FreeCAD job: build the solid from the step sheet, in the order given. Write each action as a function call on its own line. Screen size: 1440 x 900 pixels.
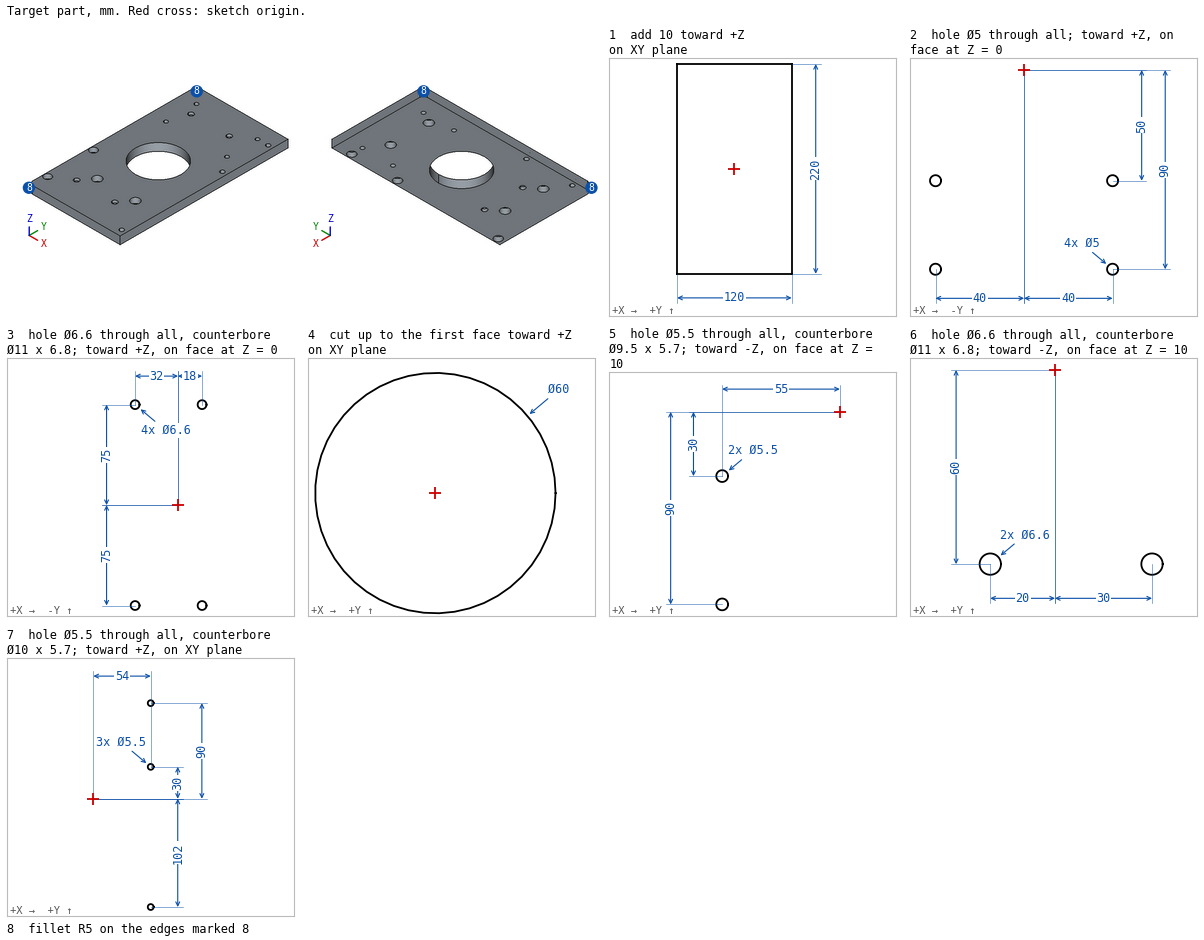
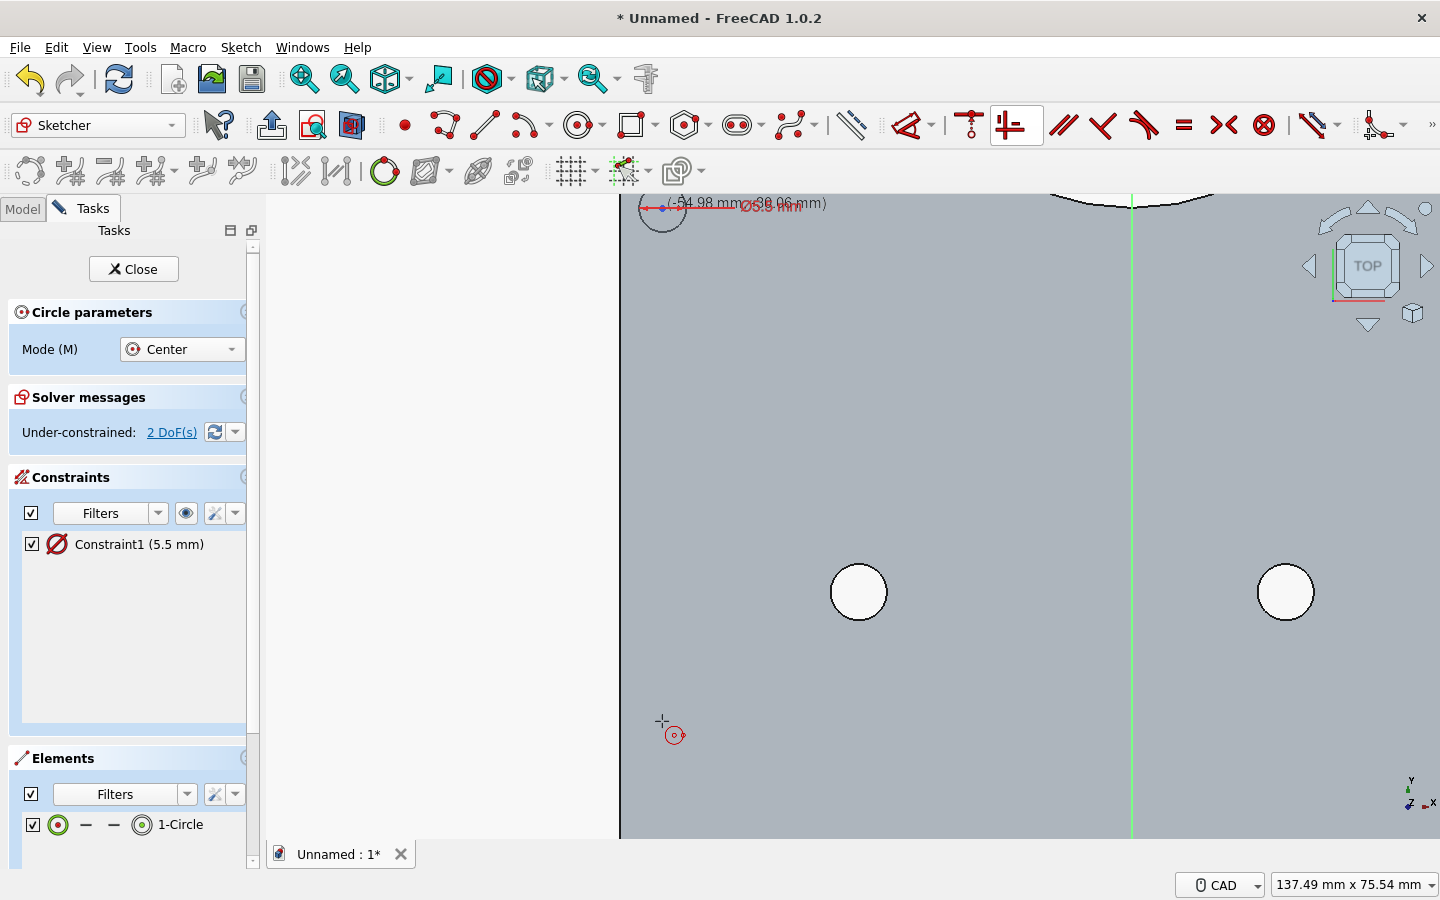
click(662, 720)
move(679, 704)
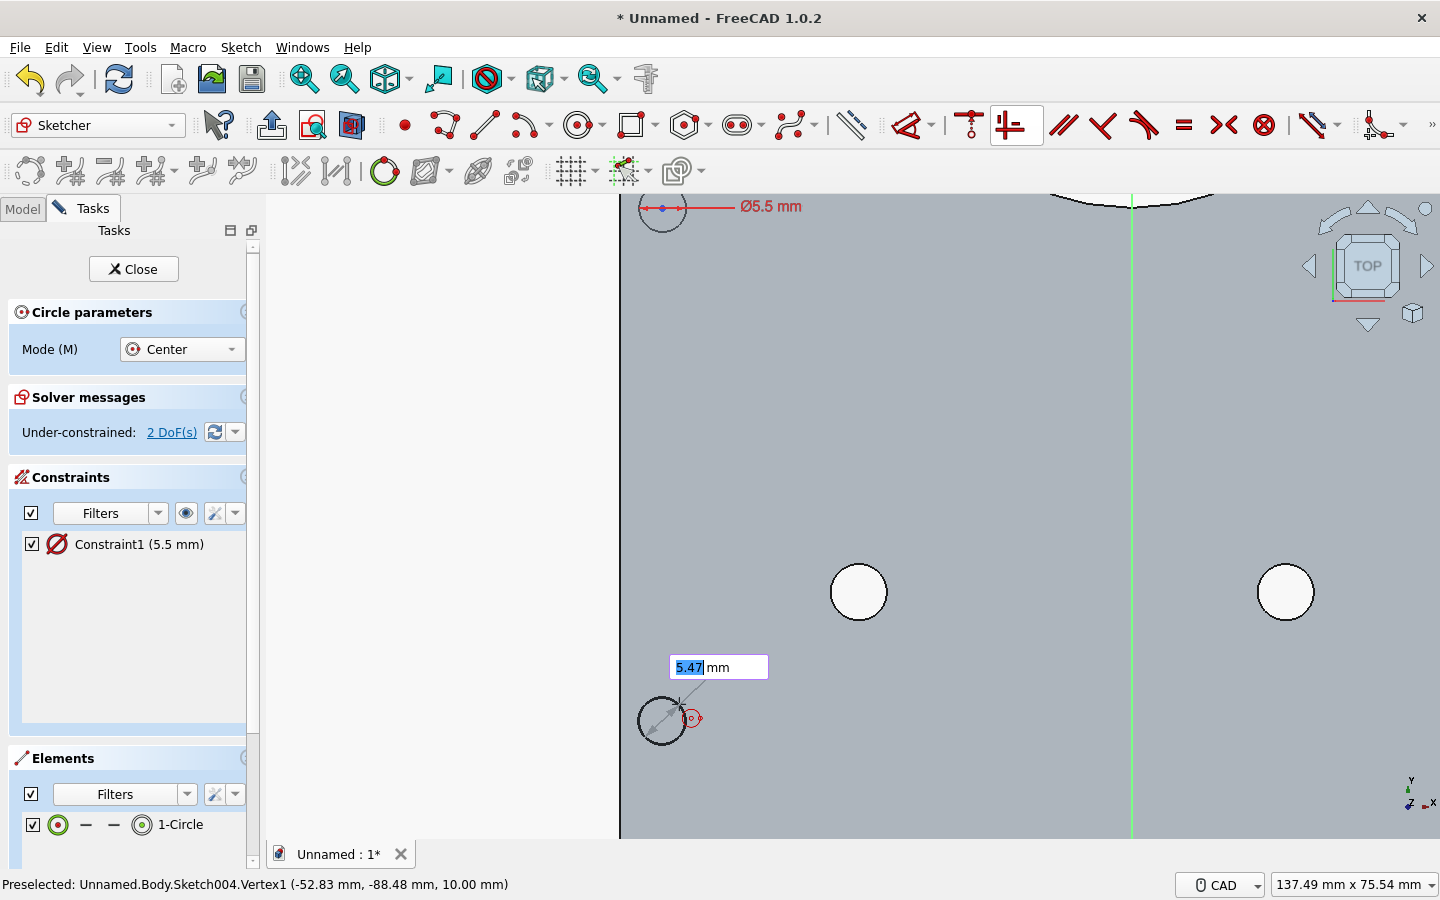
text(5.5)
key(Return)
key(Escape)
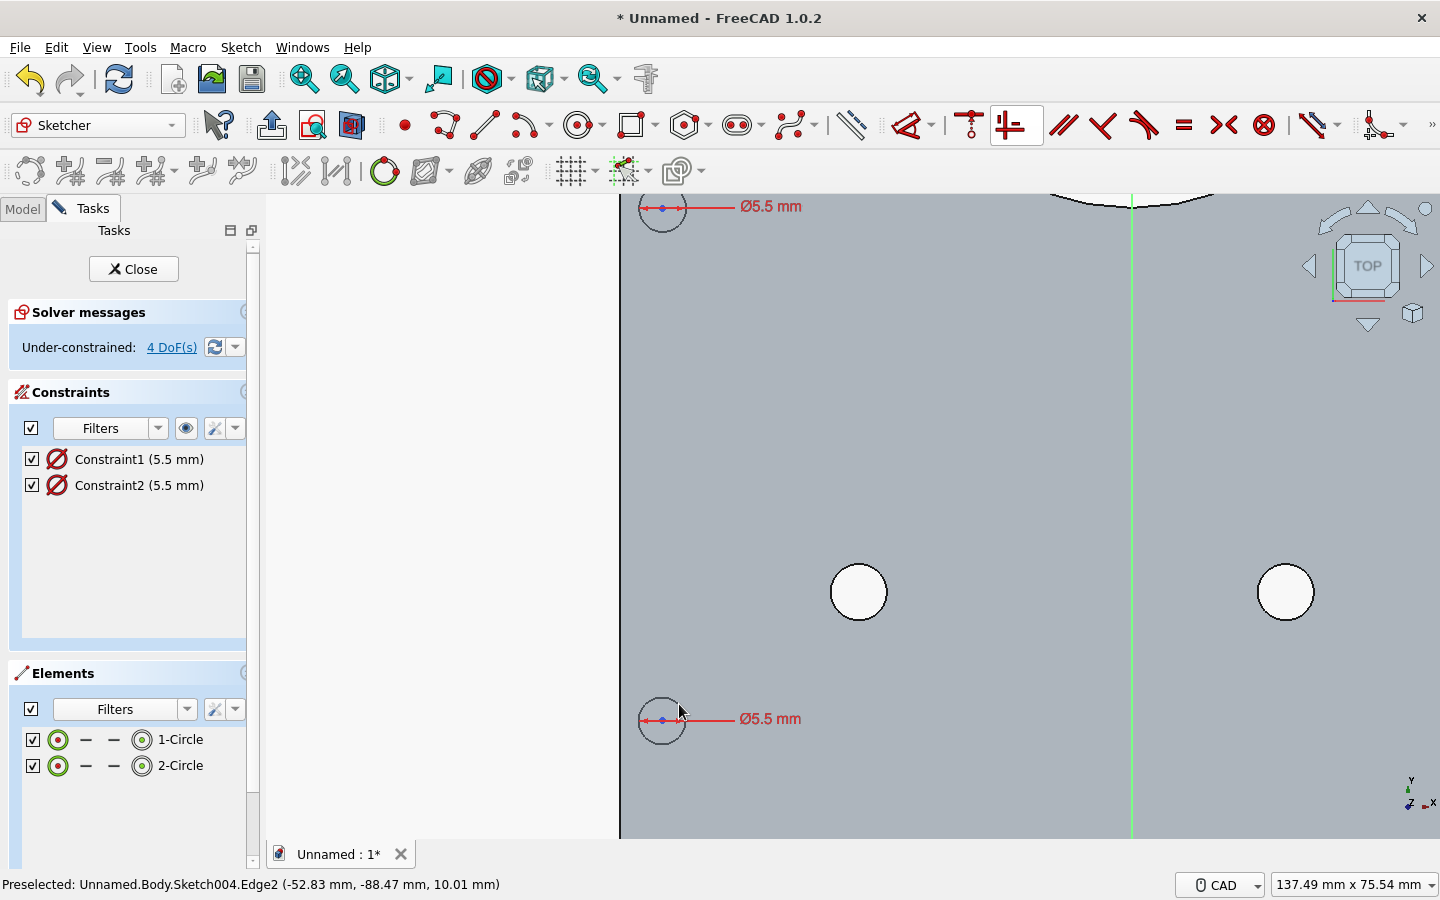
scroll(662, 722, down, 3)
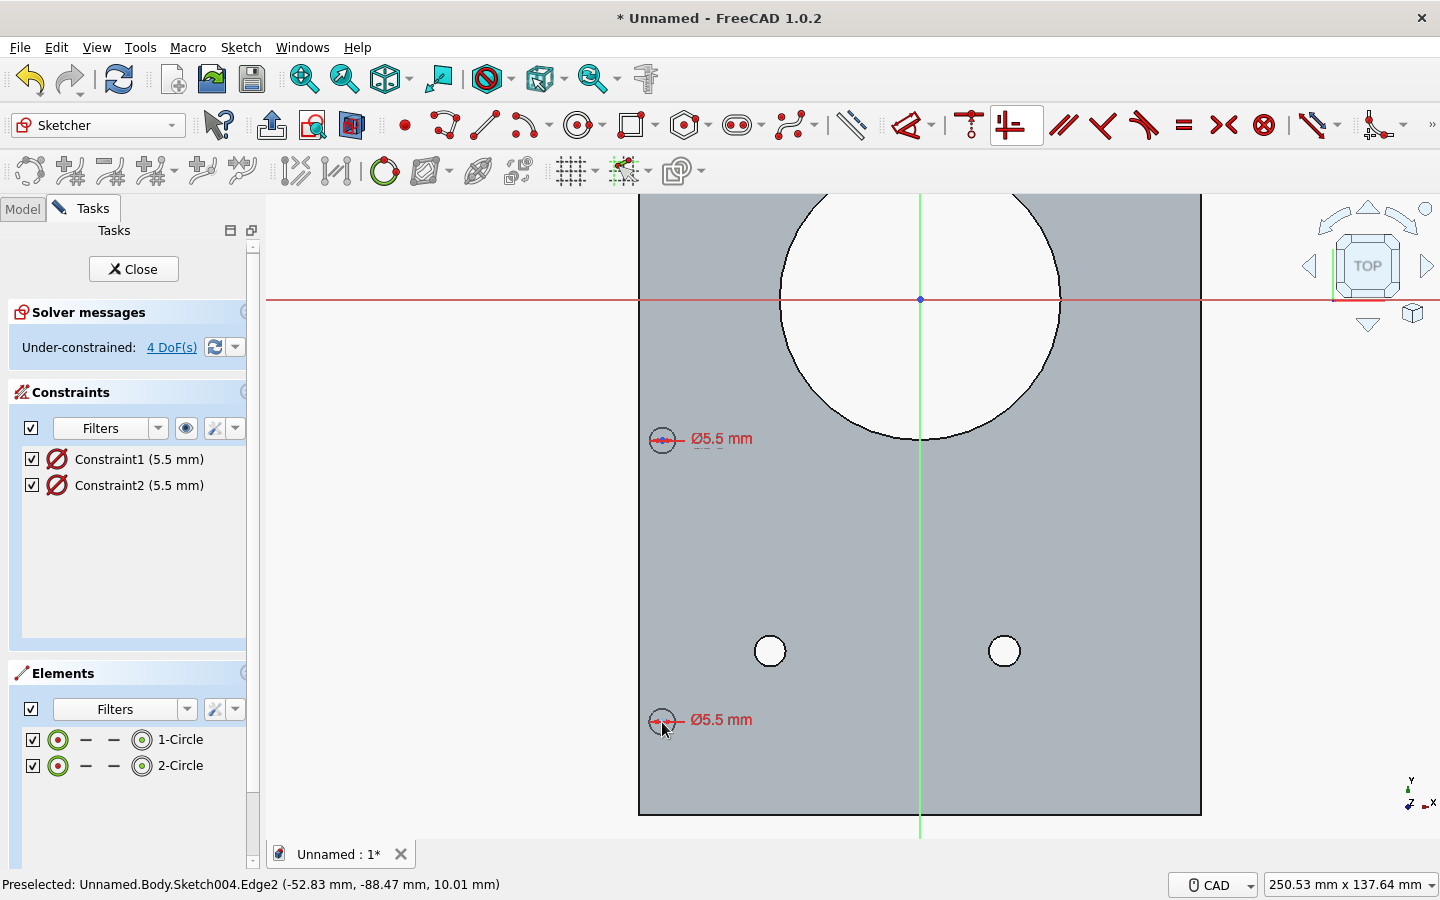
click(663, 441)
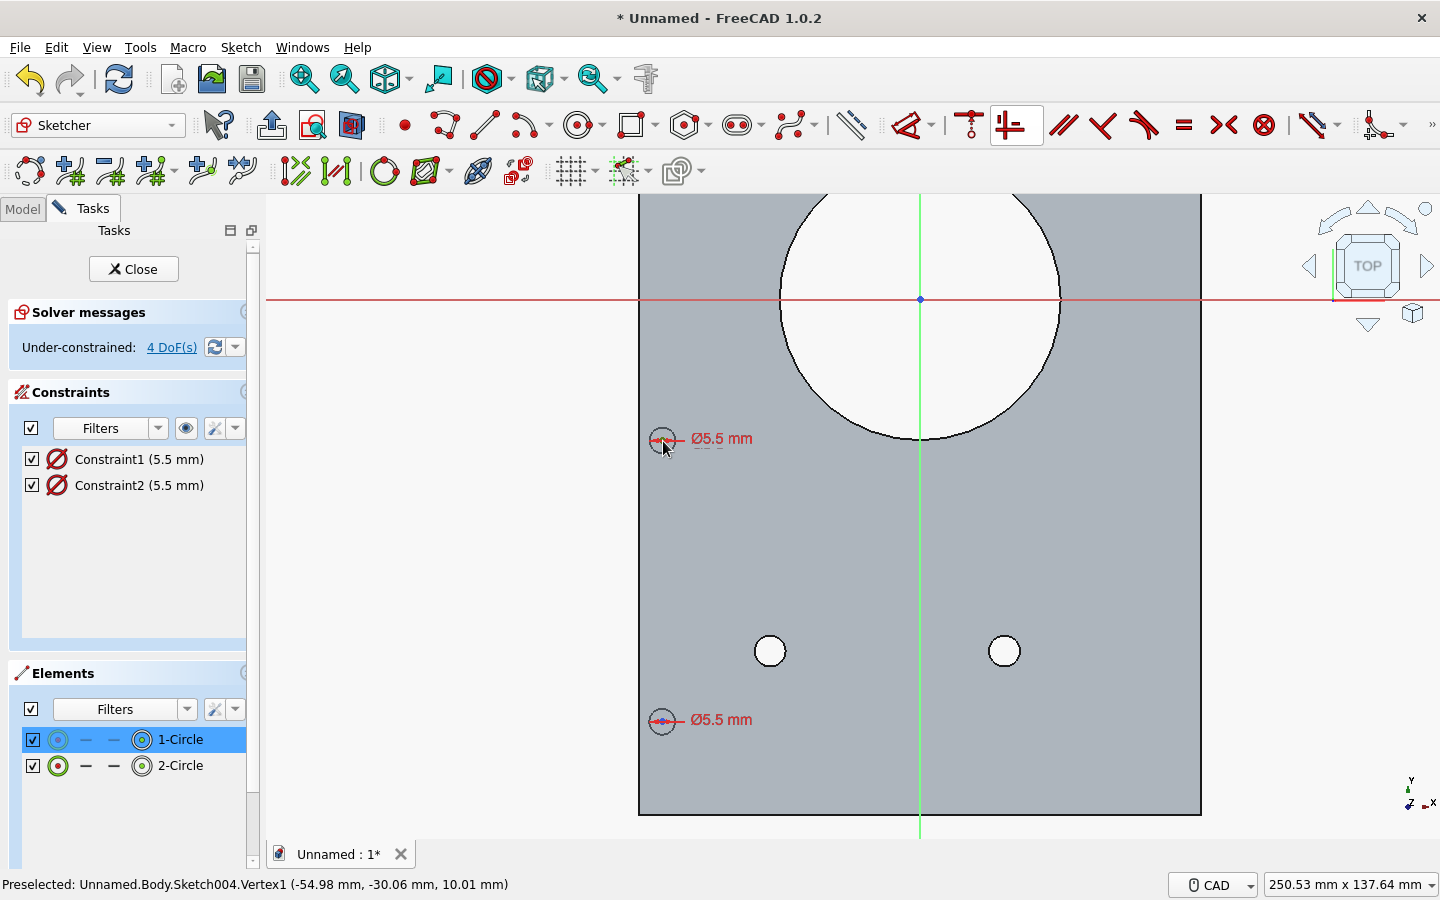
click(662, 722)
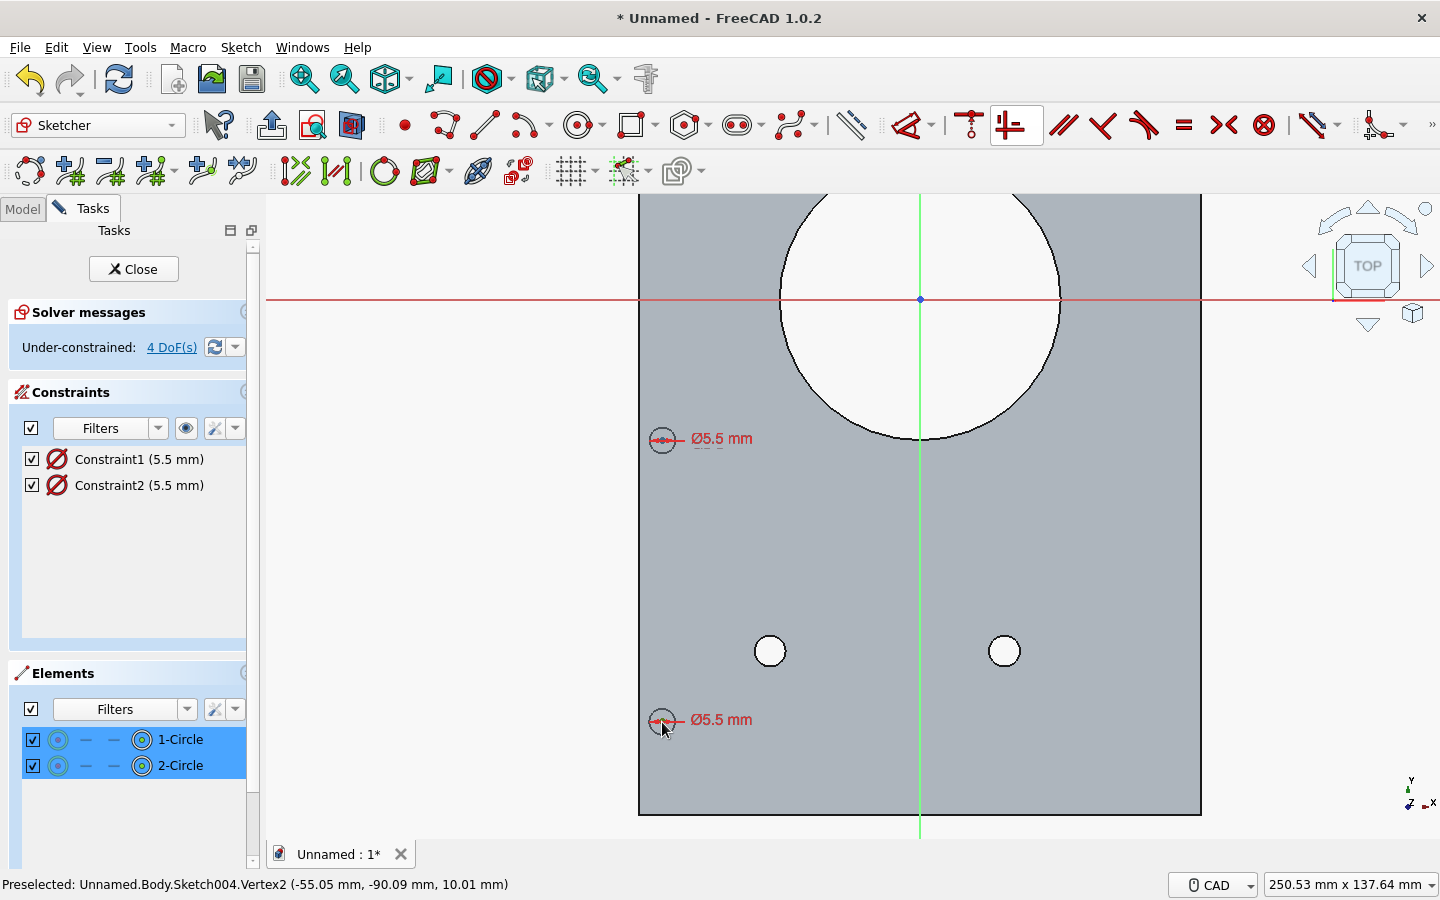
key(v)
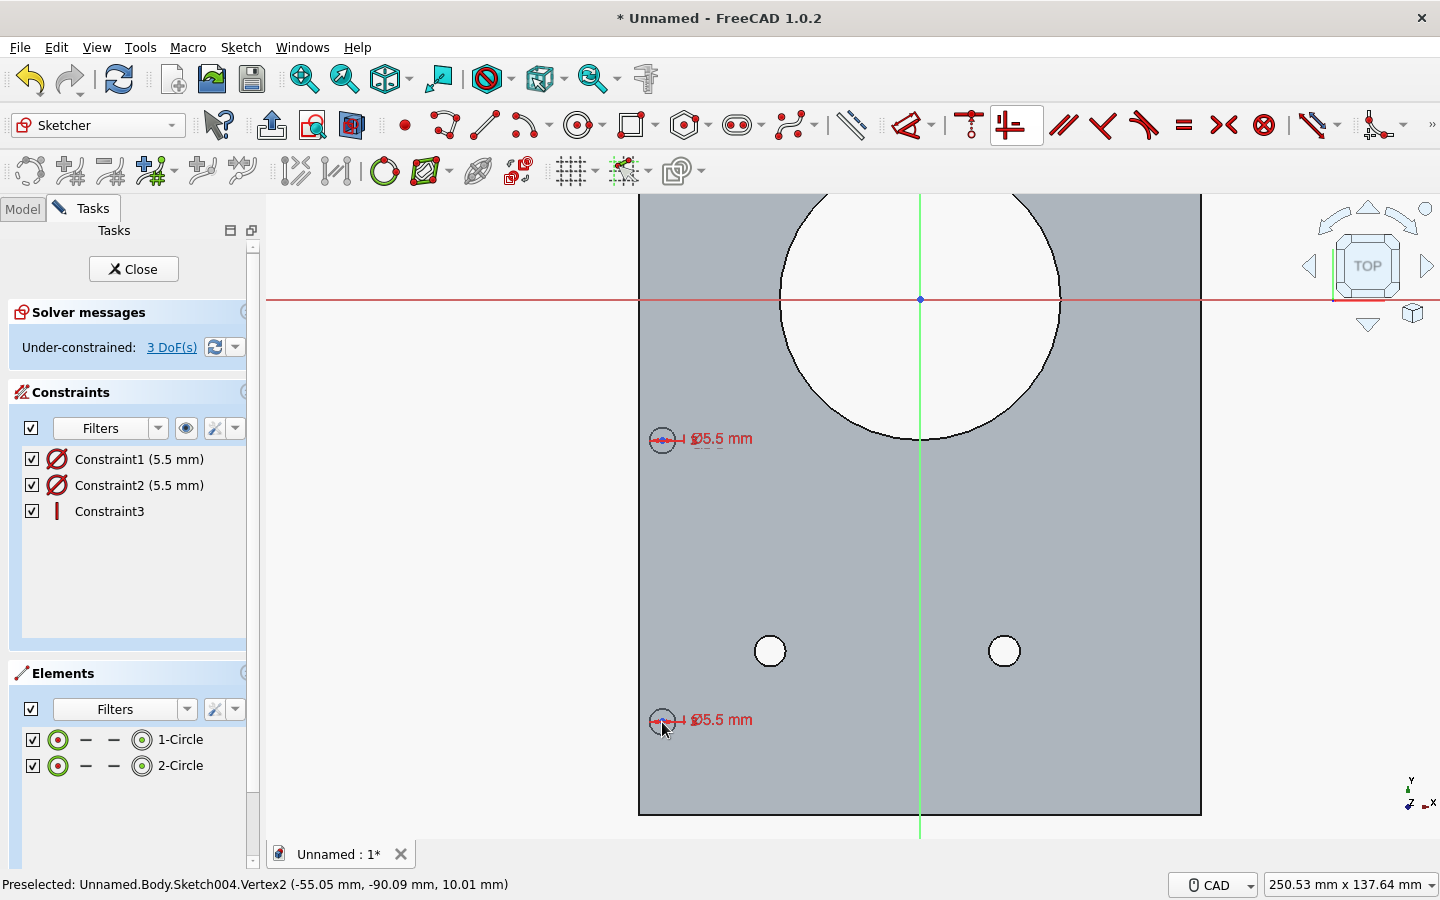
key(d)